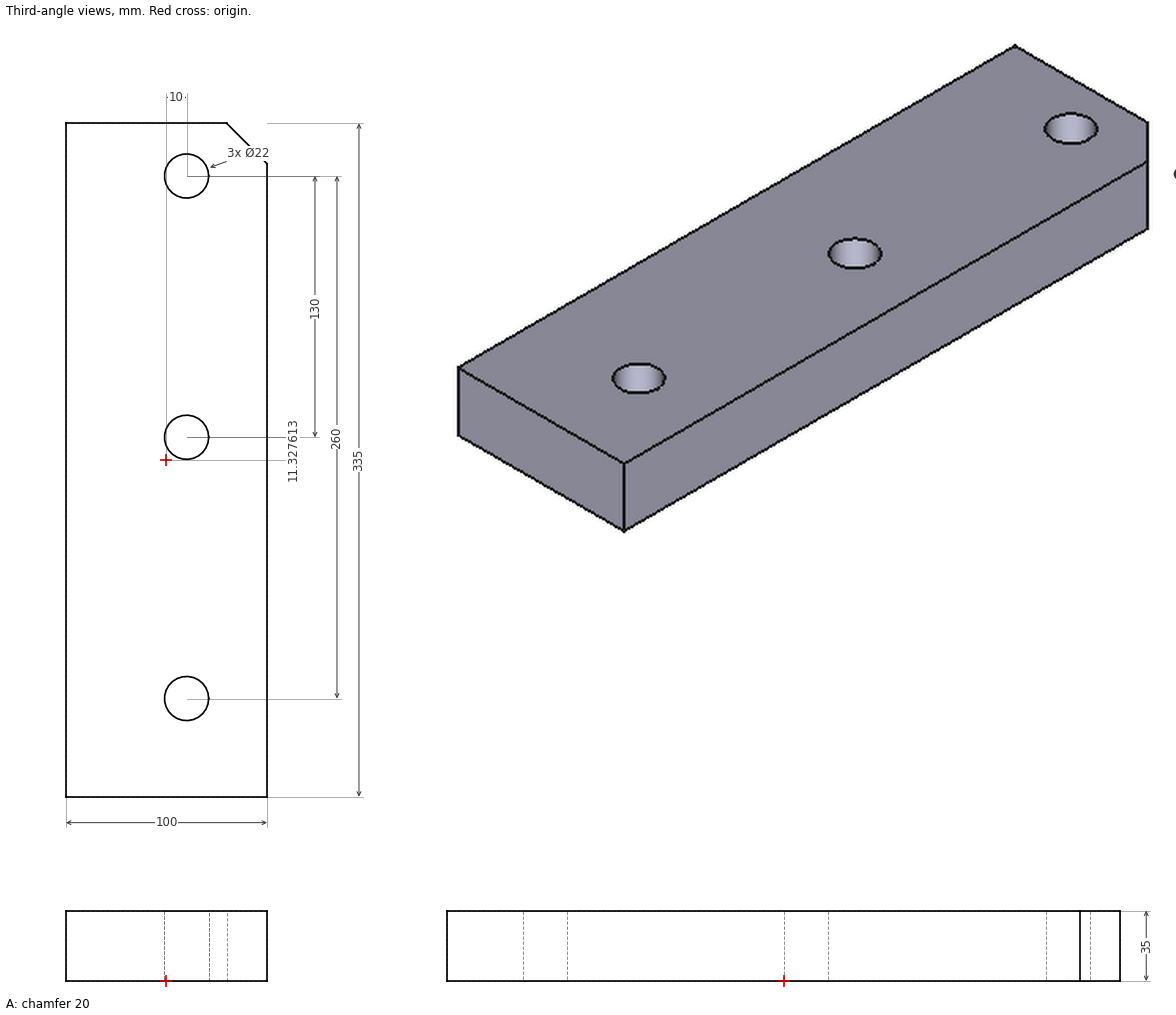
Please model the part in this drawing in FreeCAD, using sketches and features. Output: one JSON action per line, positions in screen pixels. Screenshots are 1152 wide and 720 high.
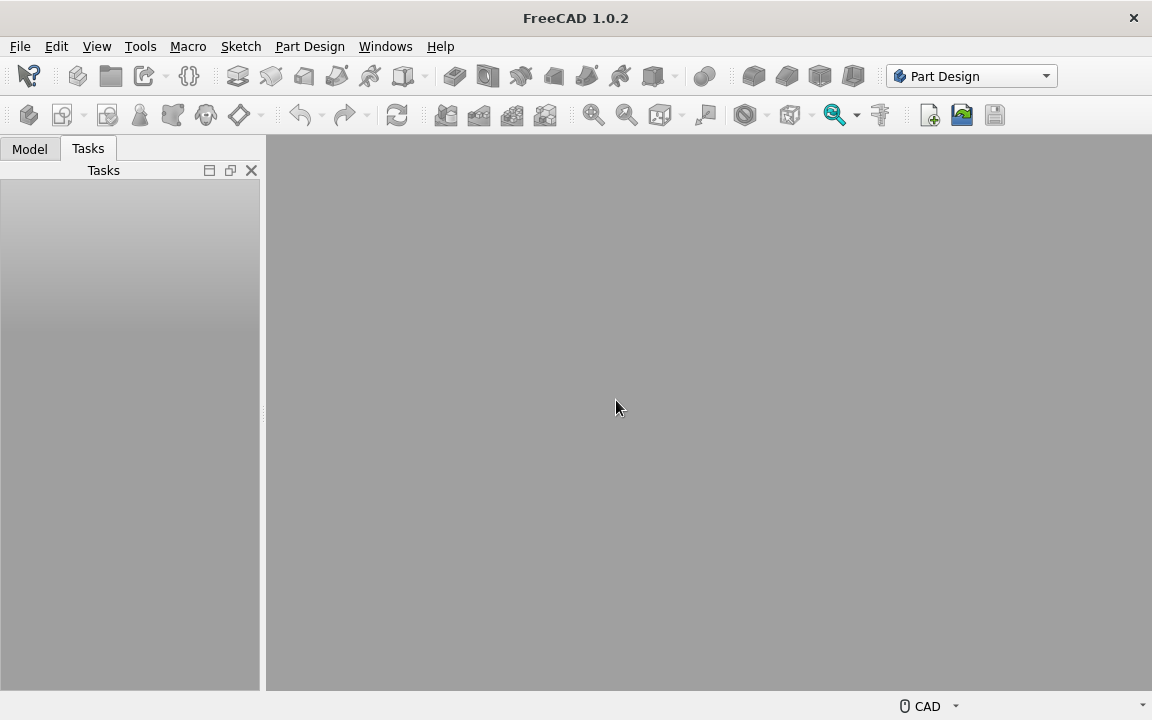
{"action": "left_click", "coordinate": [929, 116]}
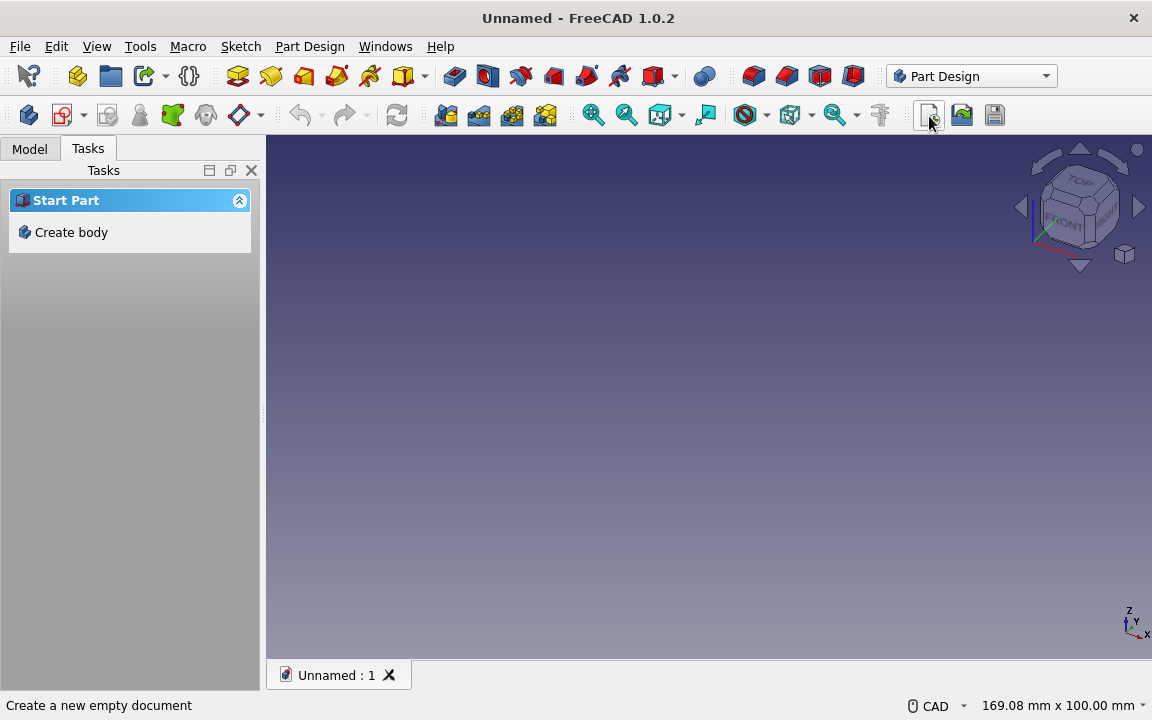
{"action": "left_click", "coordinate": [62, 116]}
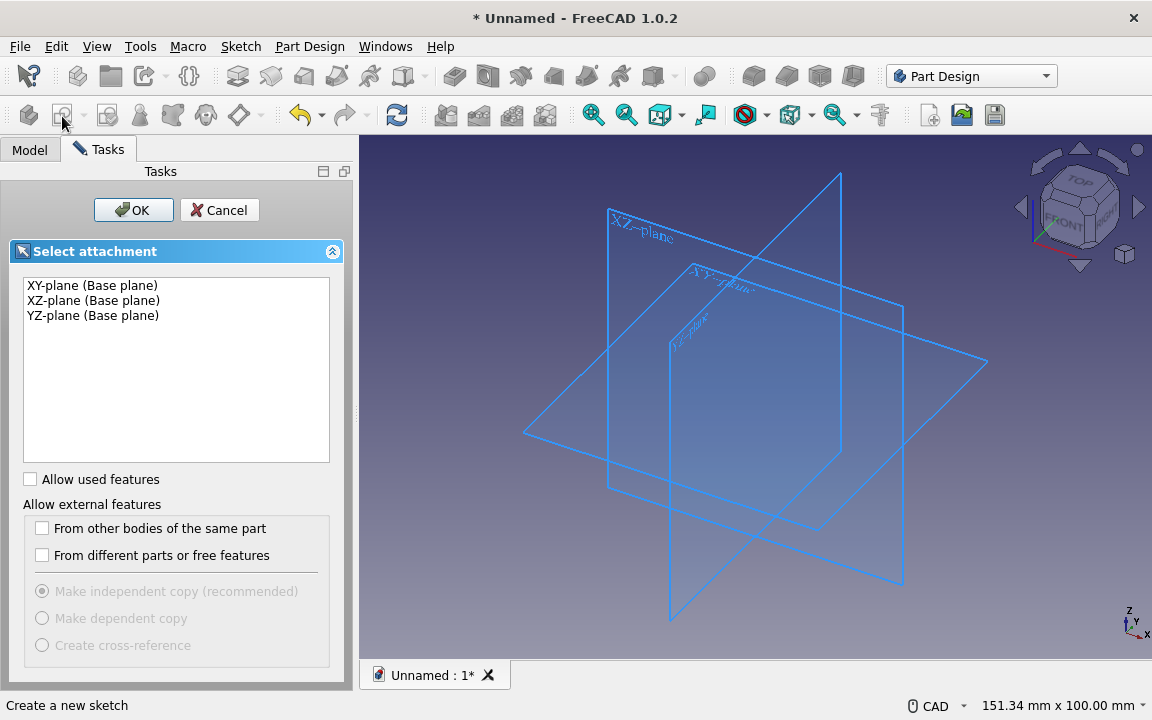
{"action": "left_click", "coordinate": [84, 286]}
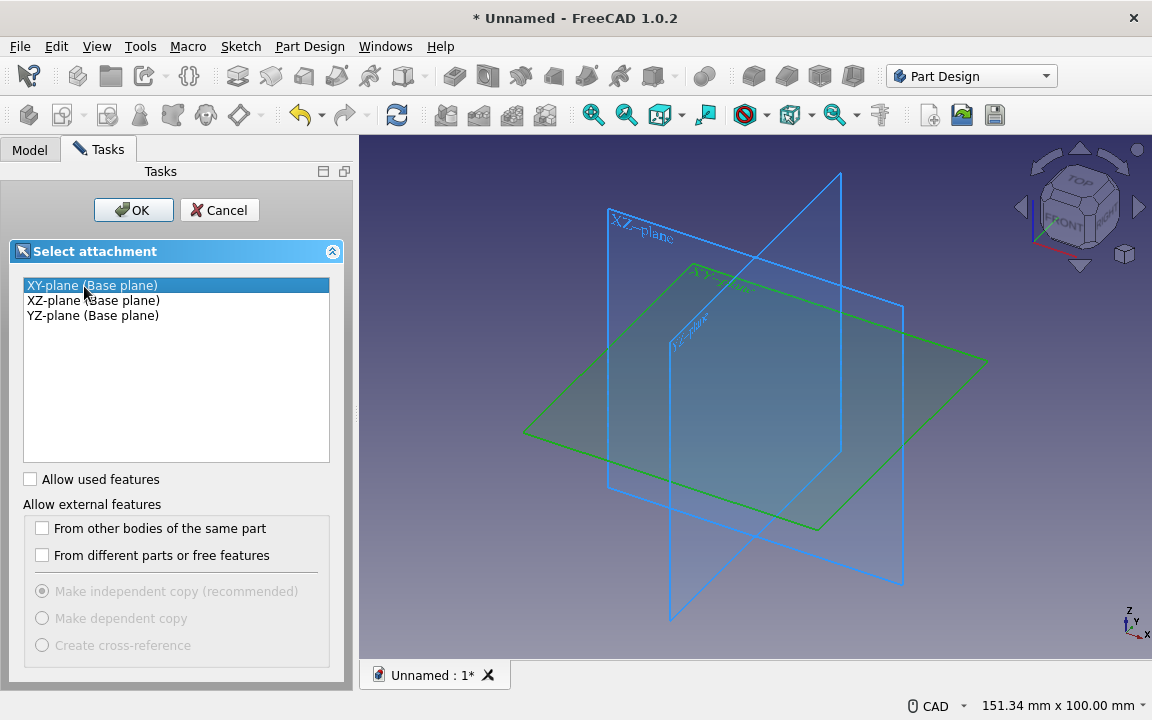
{"action": "left_click", "coordinate": [134, 210]}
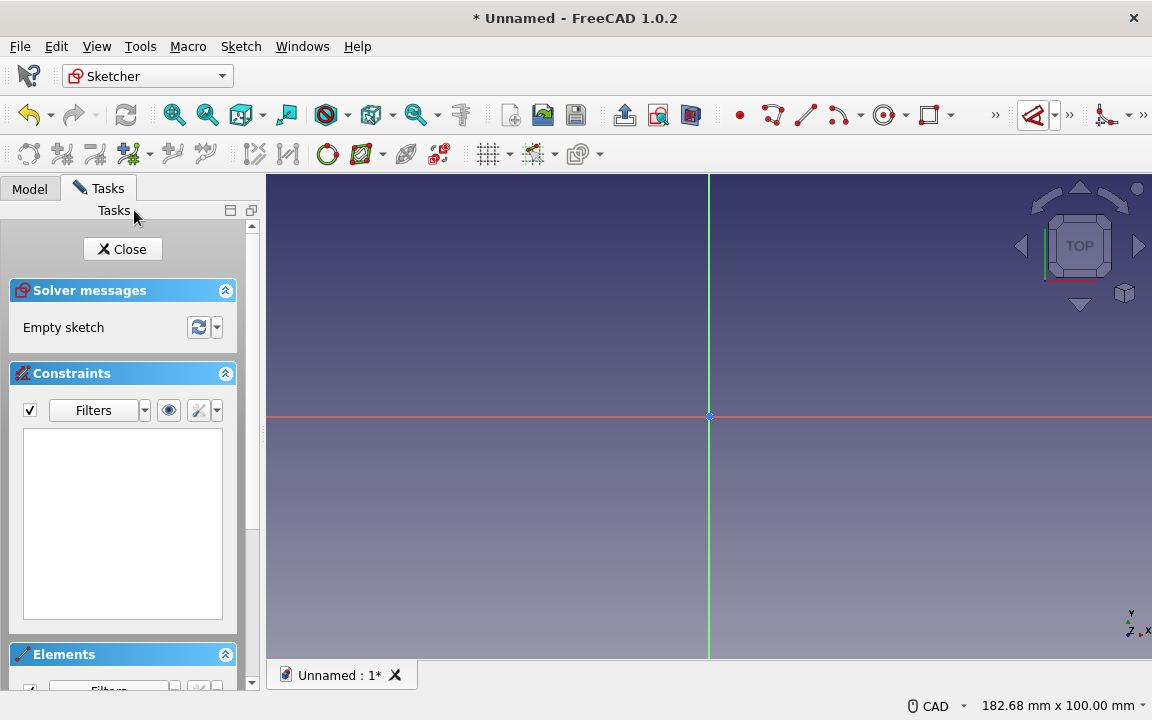
{"action": "scroll", "coordinate": [623, 416], "scroll_direction": "down", "scroll_amount": 8}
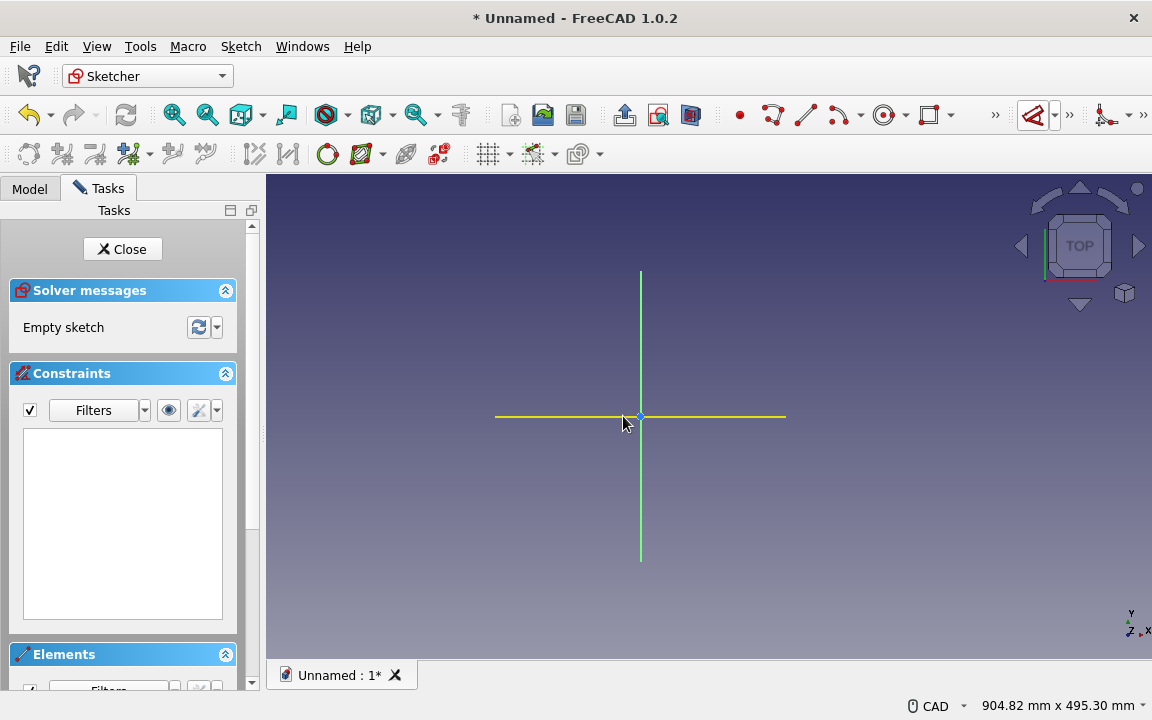
{"action": "left_click", "coordinate": [950, 116]}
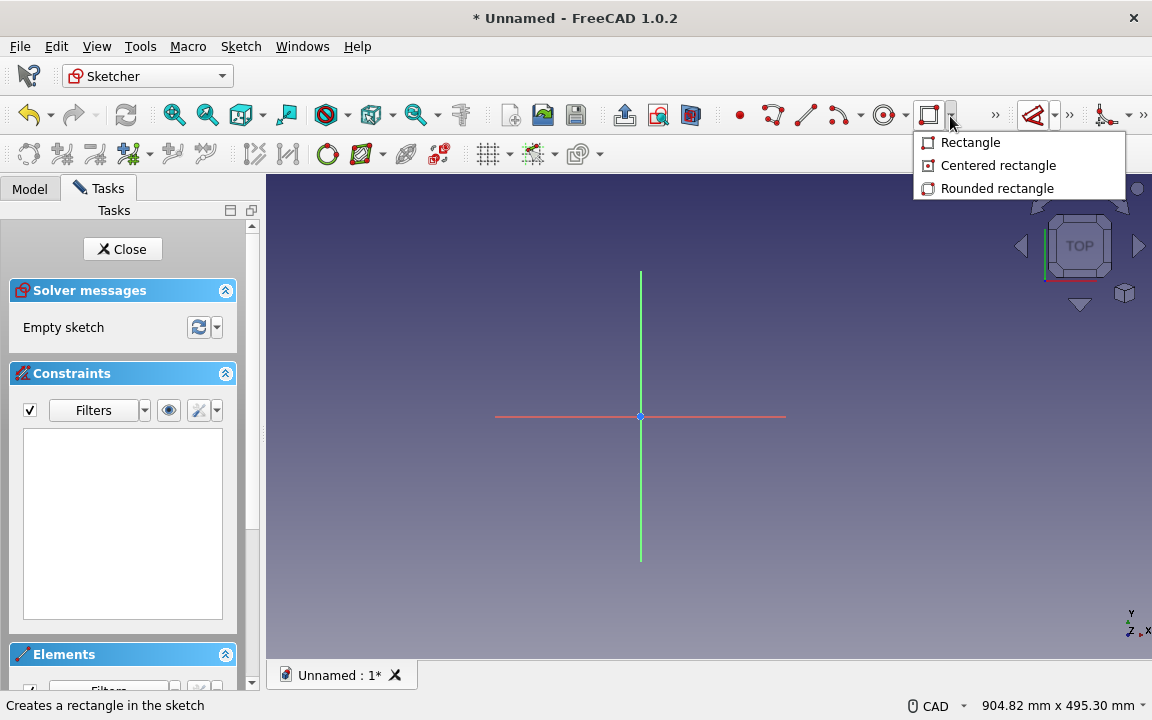
{"action": "left_click", "coordinate": [1020, 166]}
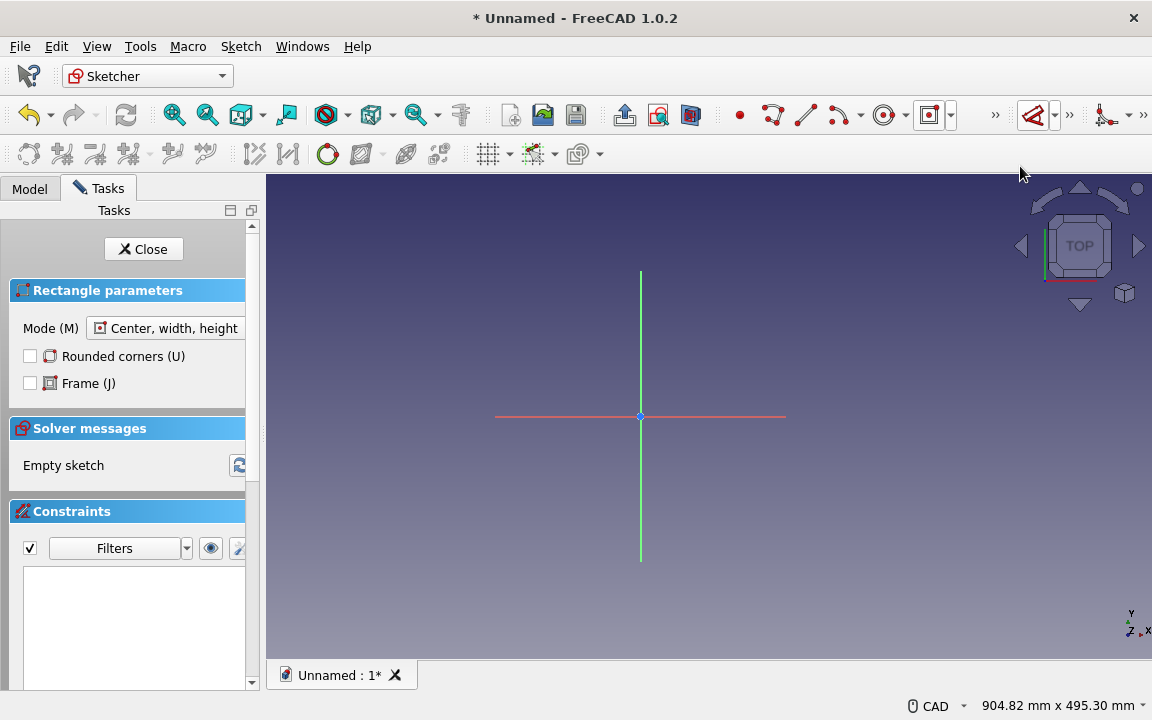
{"action": "left_click", "coordinate": [641, 416]}
{"action": "mouse_move", "coordinate": [690, 252]}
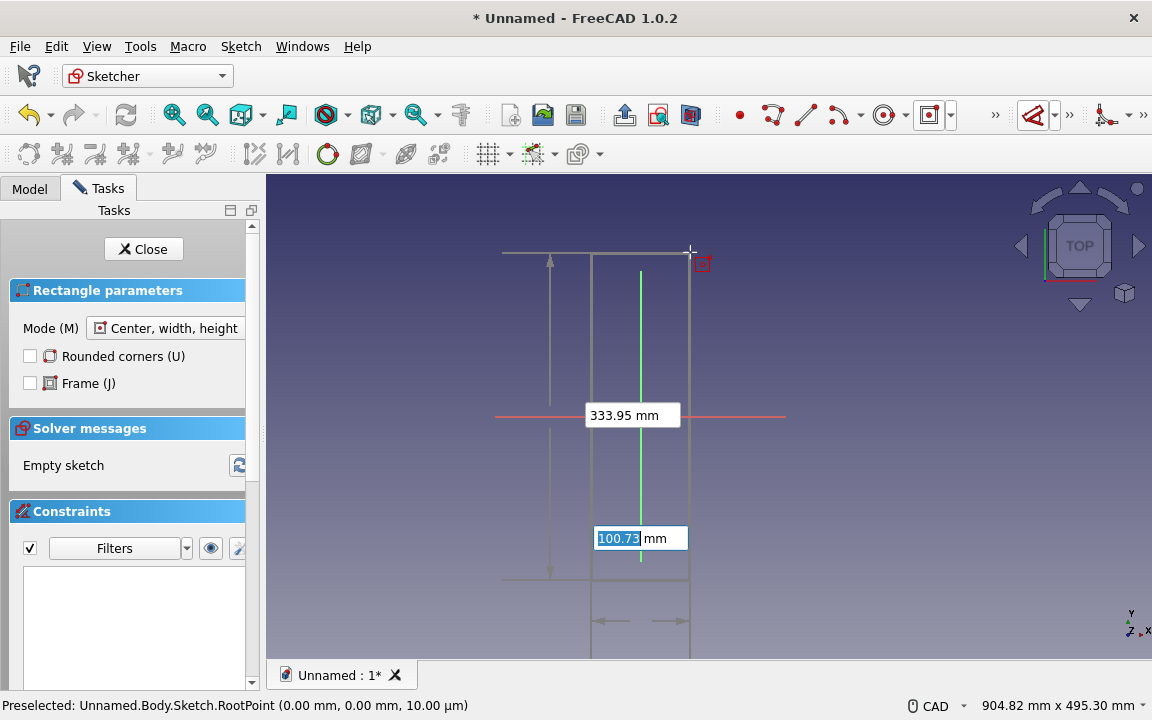
{"action": "type", "text": "100"}
{"action": "key", "text": "Tab"}
{"action": "type", "text": "335"}
{"action": "key", "text": "Return"}
{"action": "key", "text": "Escape"}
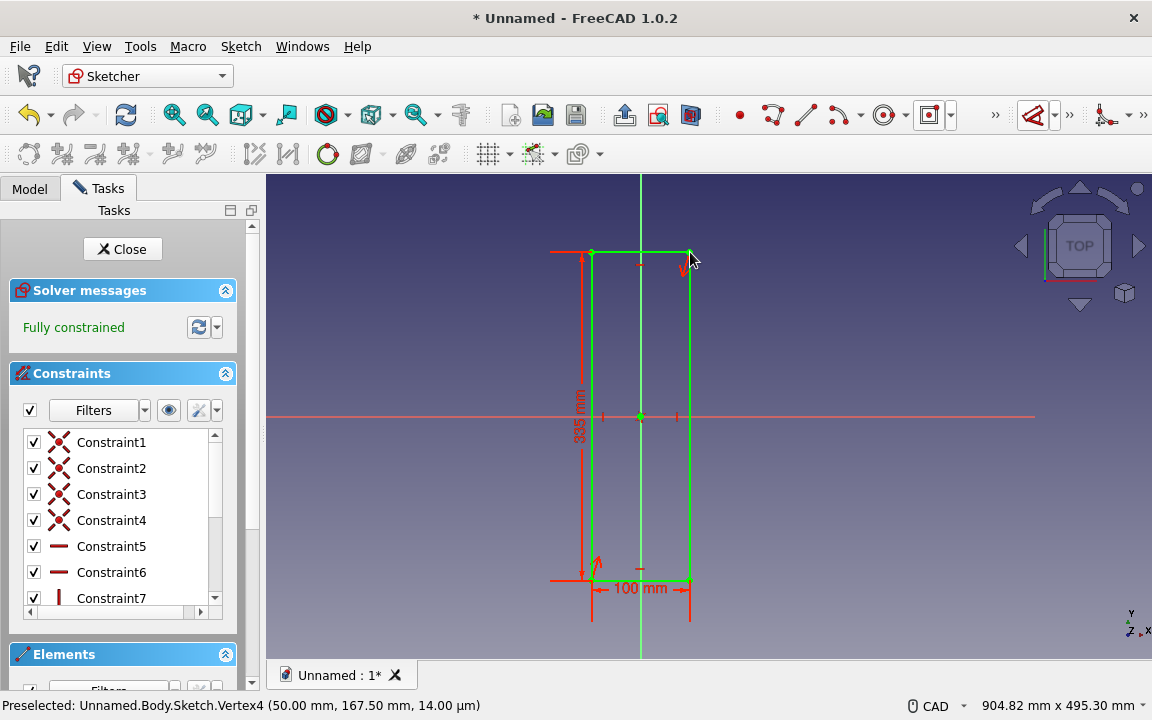
{"action": "left_click", "coordinate": [123, 249]}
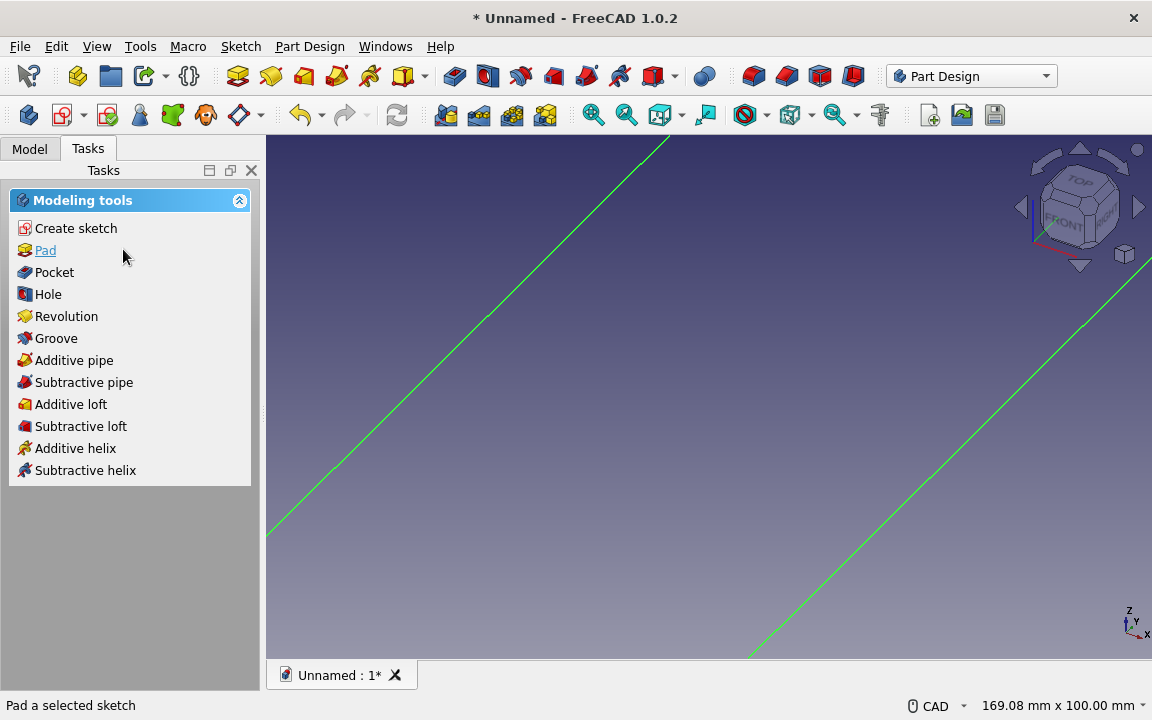
{"action": "left_click", "coordinate": [238, 76]}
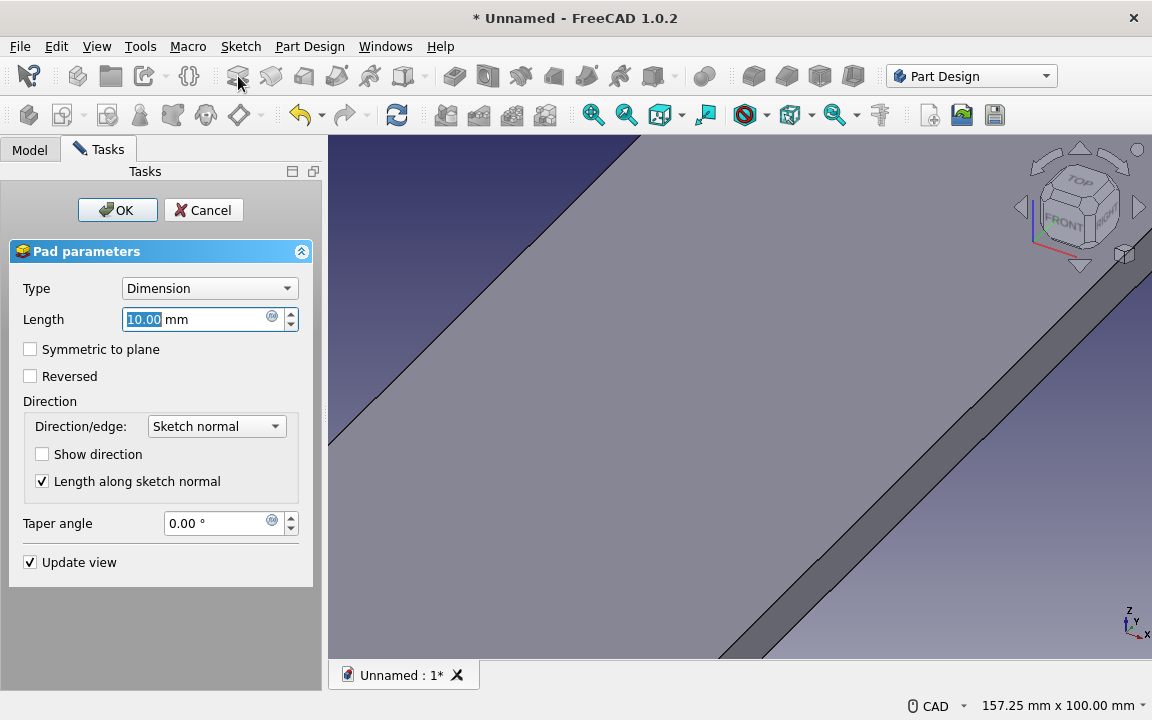
{"action": "type", "text": "35"}
{"action": "key", "text": "Tab"}